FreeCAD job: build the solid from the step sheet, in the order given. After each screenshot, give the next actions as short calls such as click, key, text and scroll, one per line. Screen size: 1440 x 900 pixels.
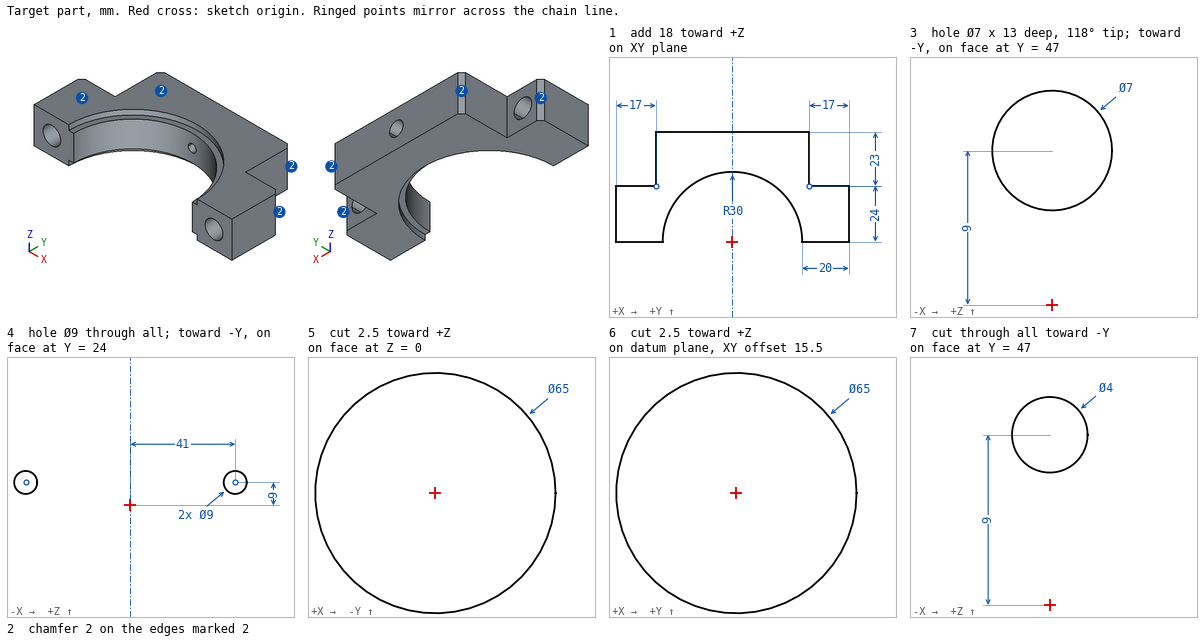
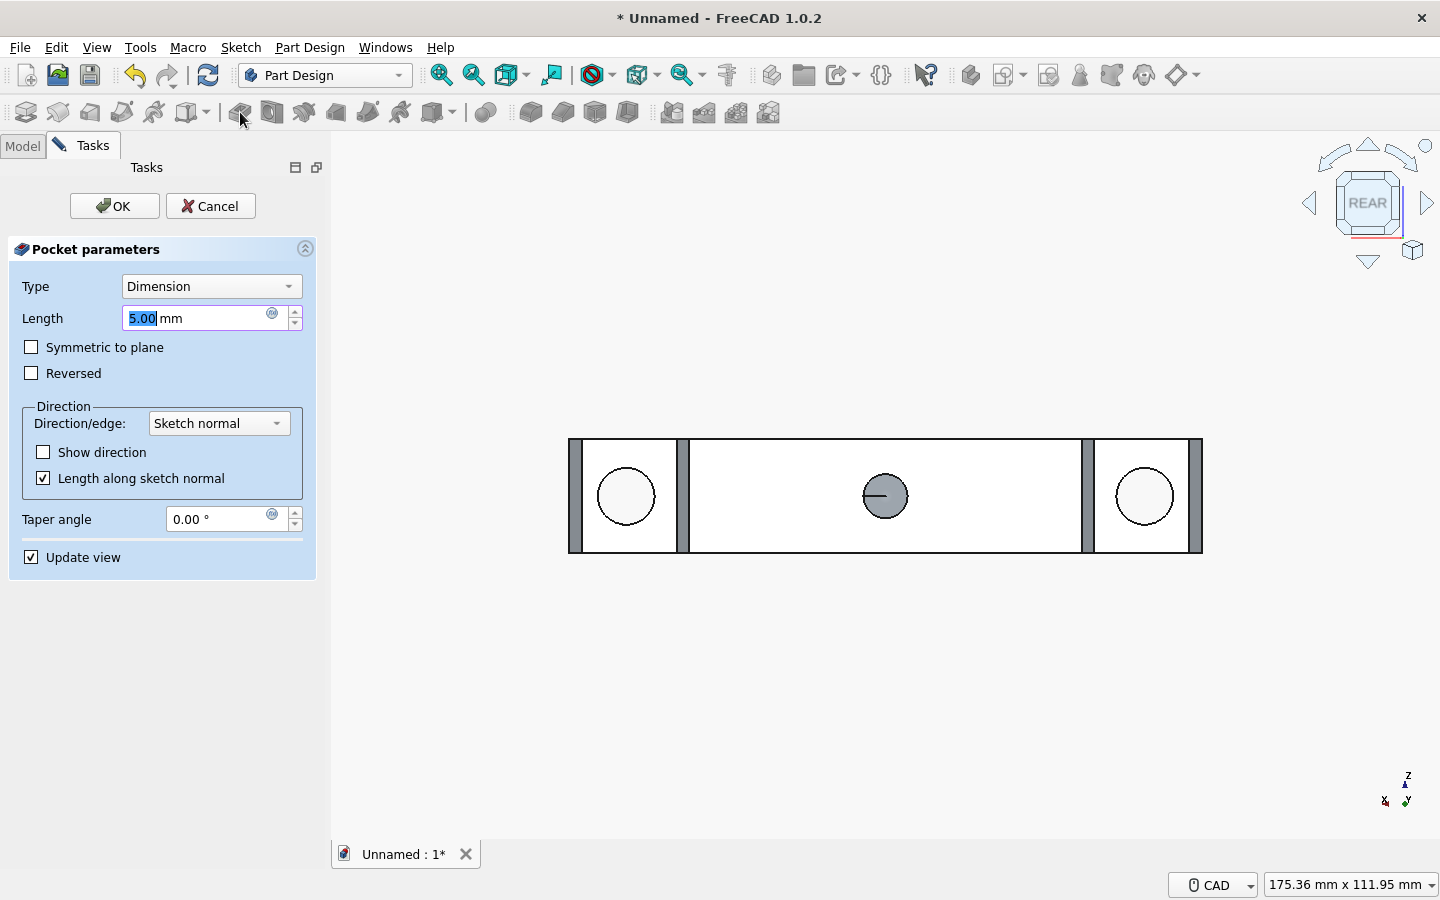
click(212, 286)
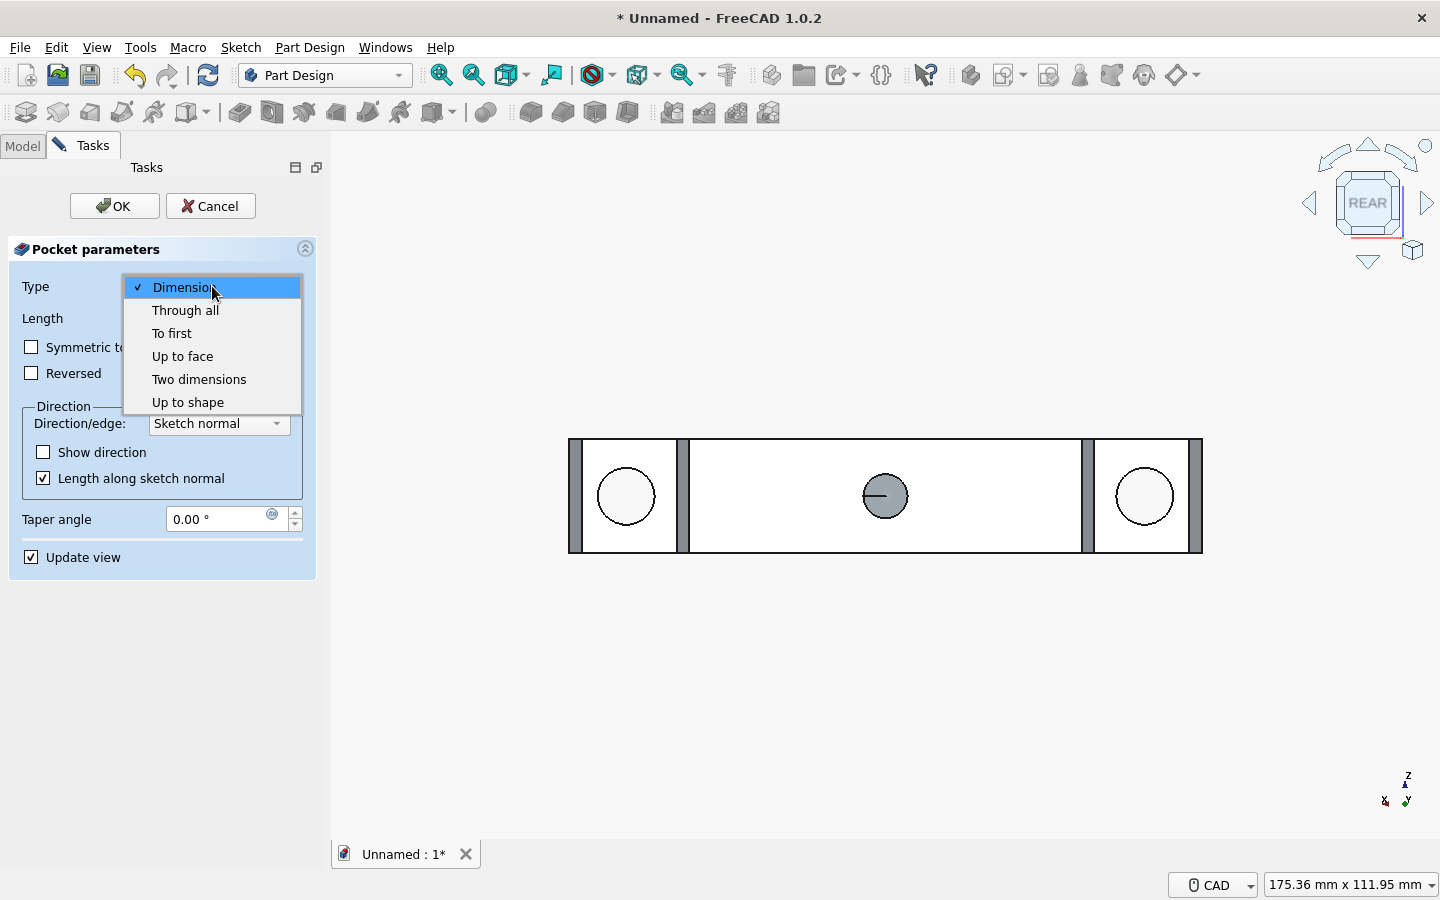
click(212, 310)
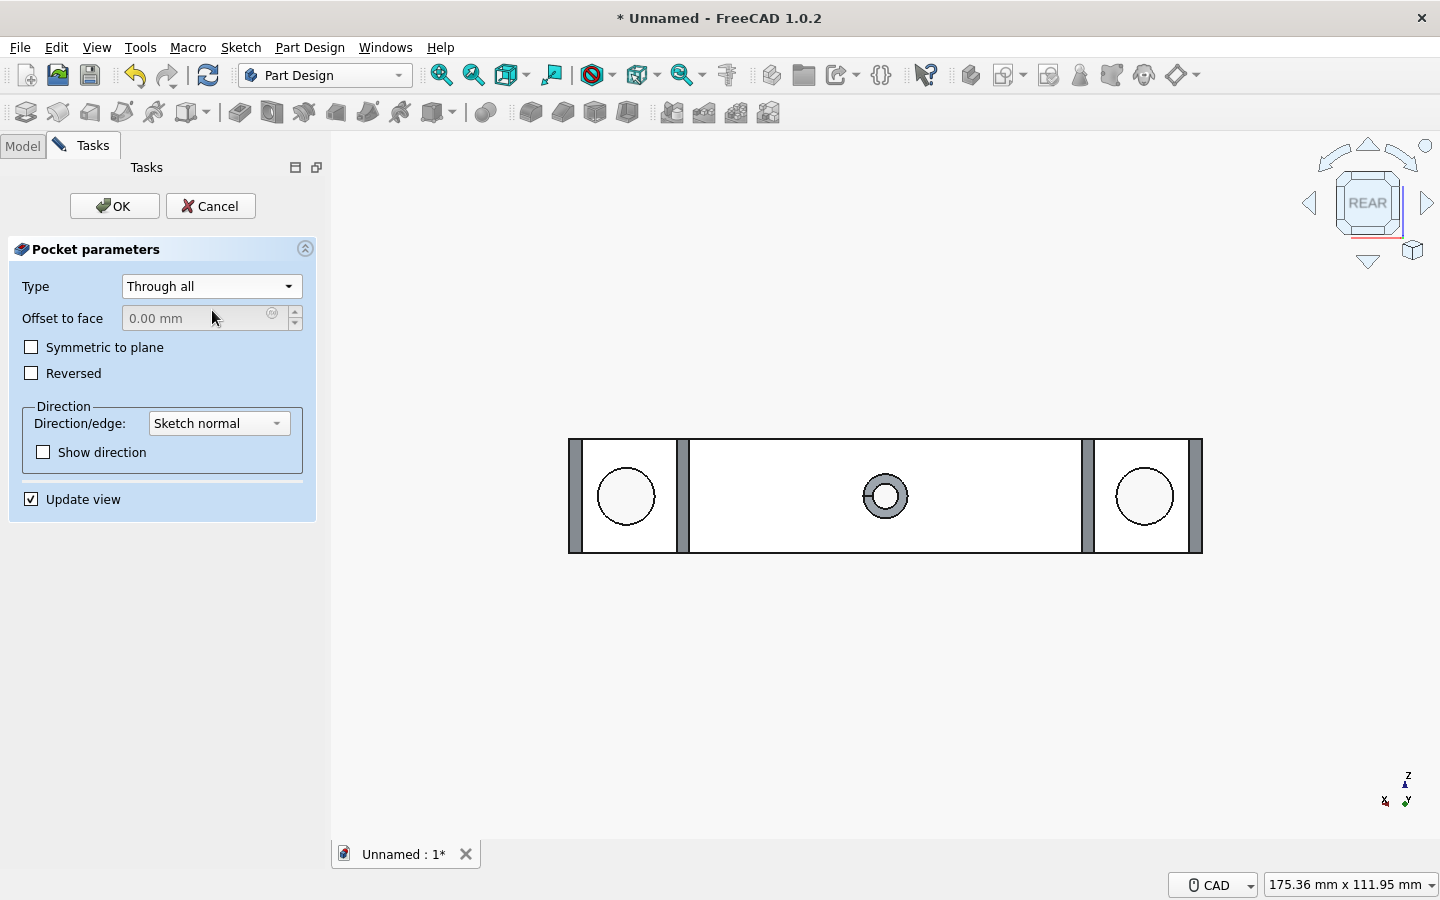
click(115, 206)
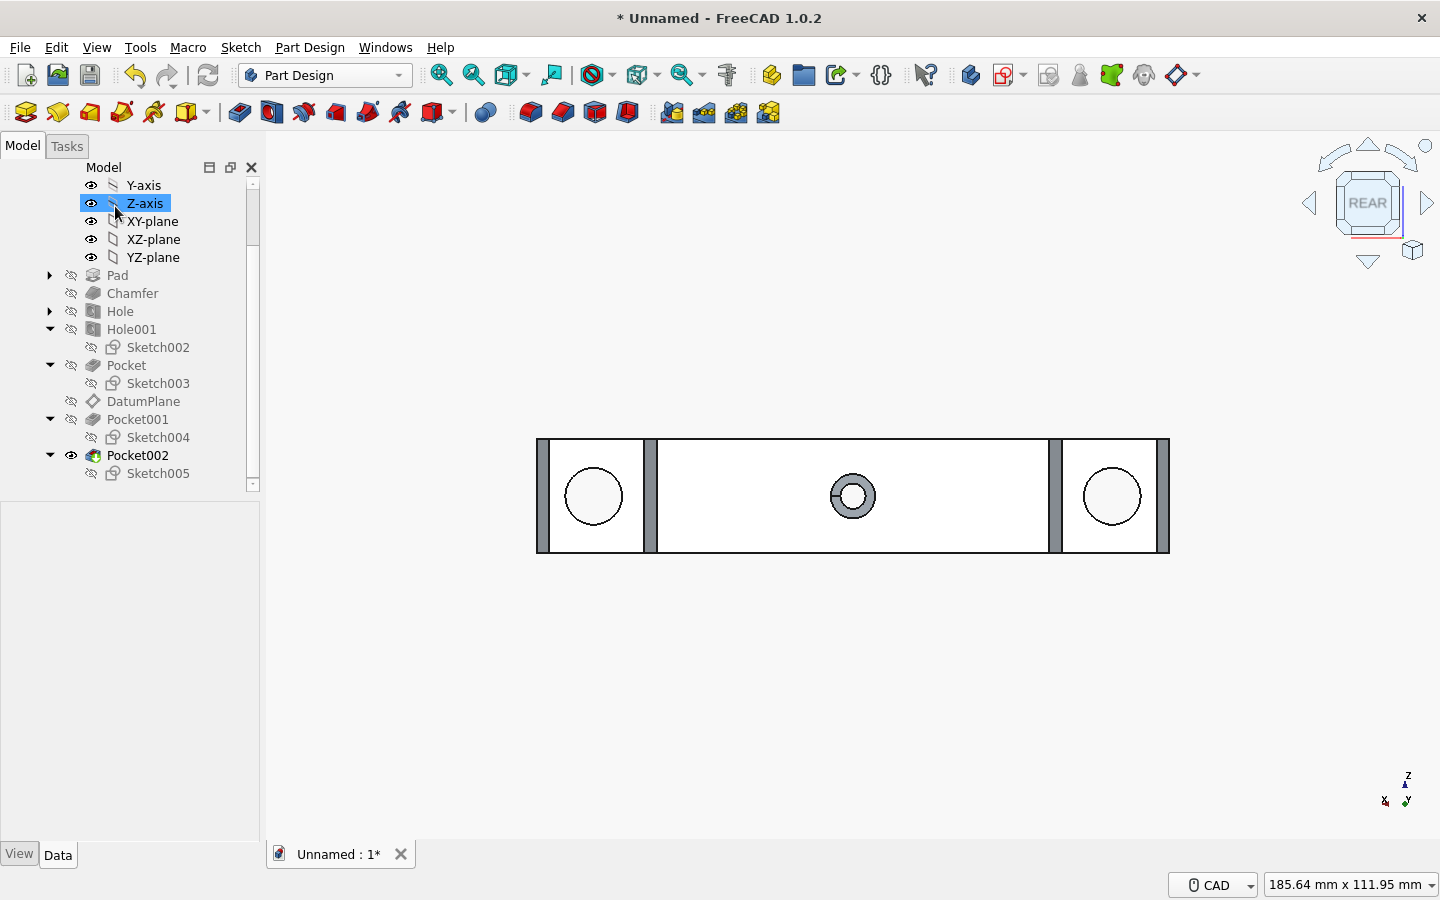
key(0)